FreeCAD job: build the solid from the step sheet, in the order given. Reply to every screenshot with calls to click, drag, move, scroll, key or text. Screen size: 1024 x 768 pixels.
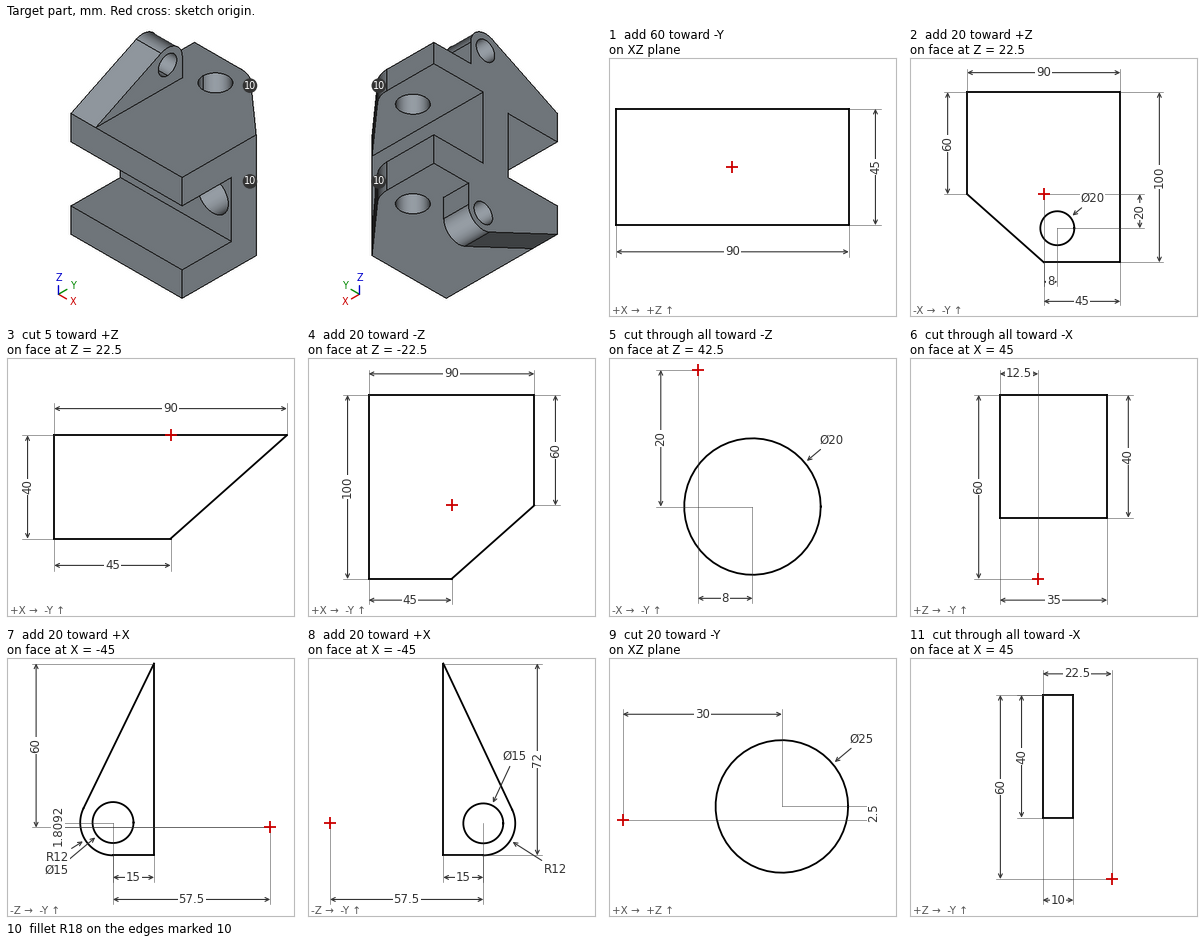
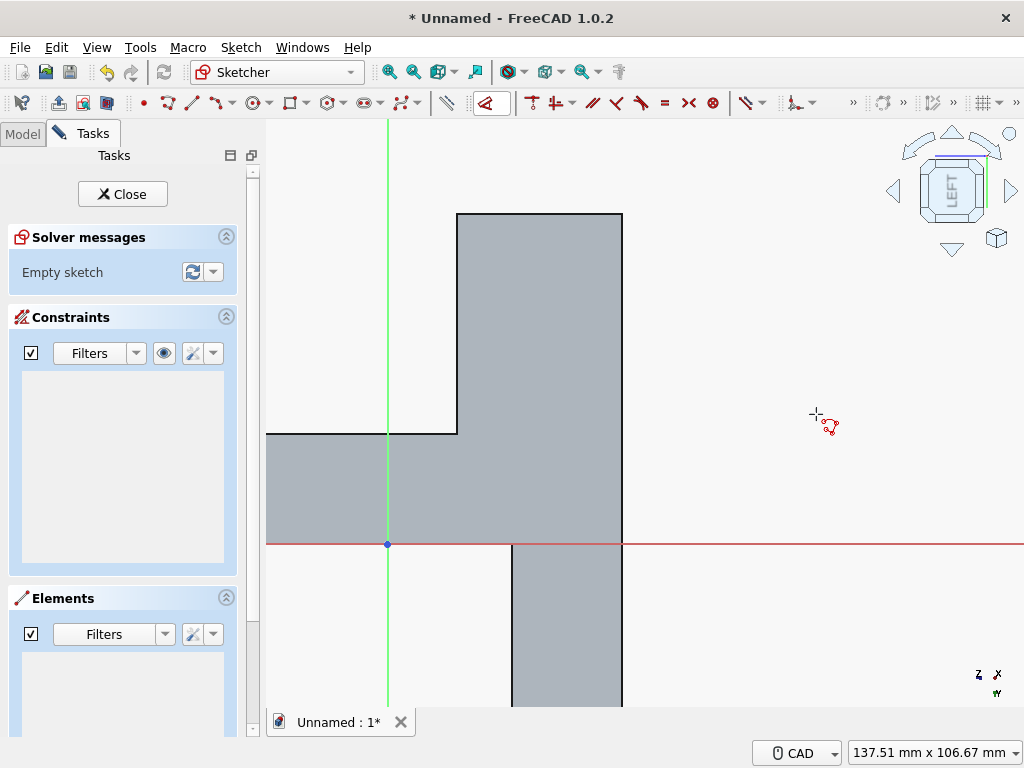
click(765, 516)
click(622, 214)
click(622, 611)
click(705, 611)
right_click(705, 611)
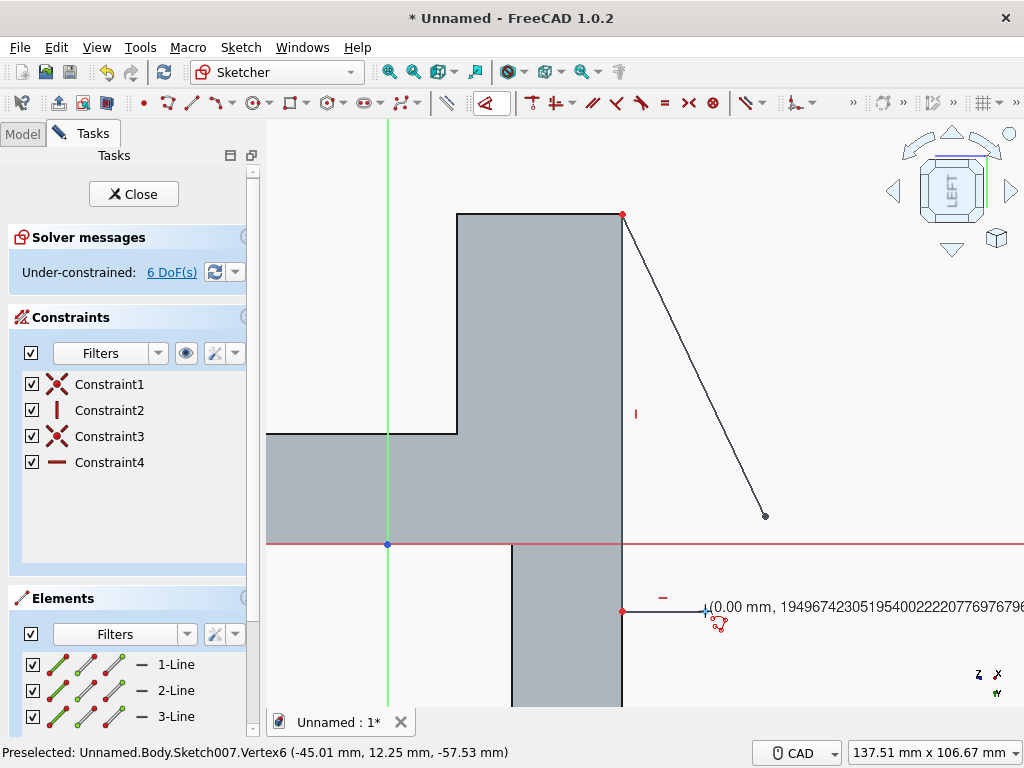
key(g)
key(3)
key(a)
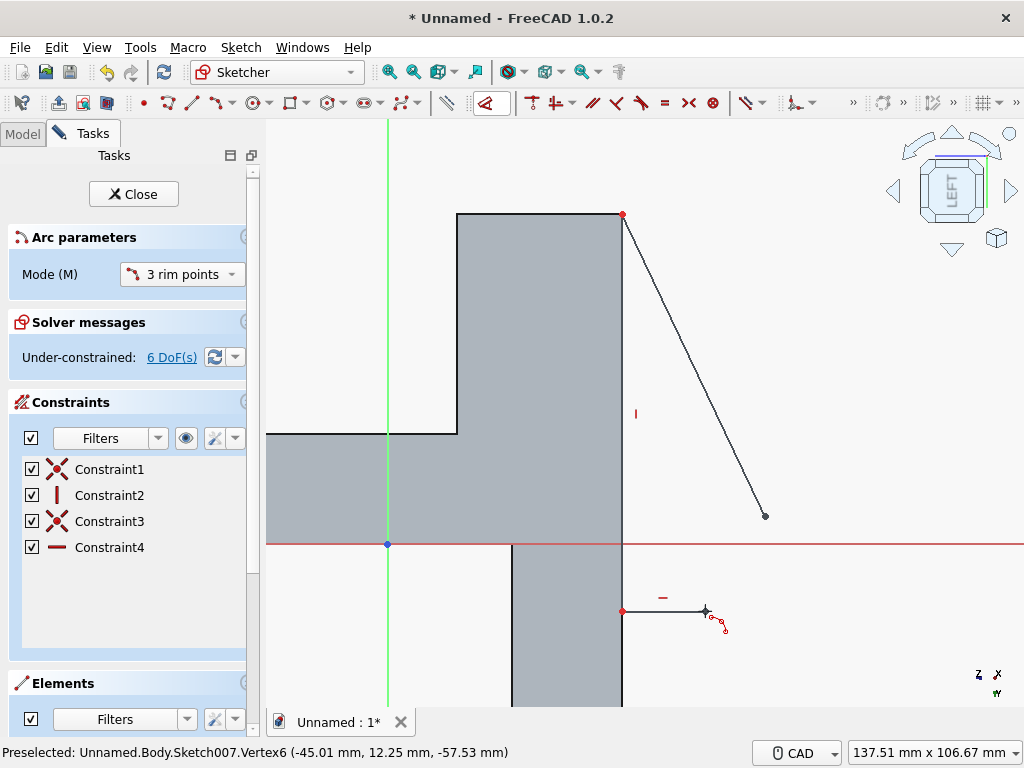
click(705, 612)
click(765, 517)
click(761, 580)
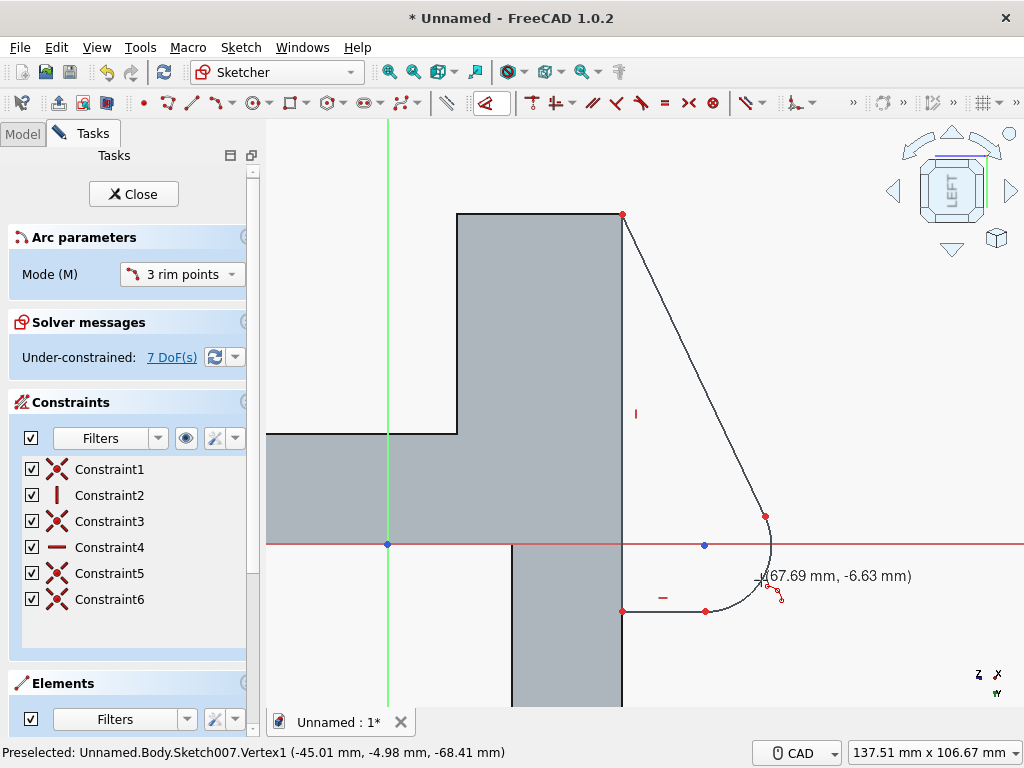
click(254, 104)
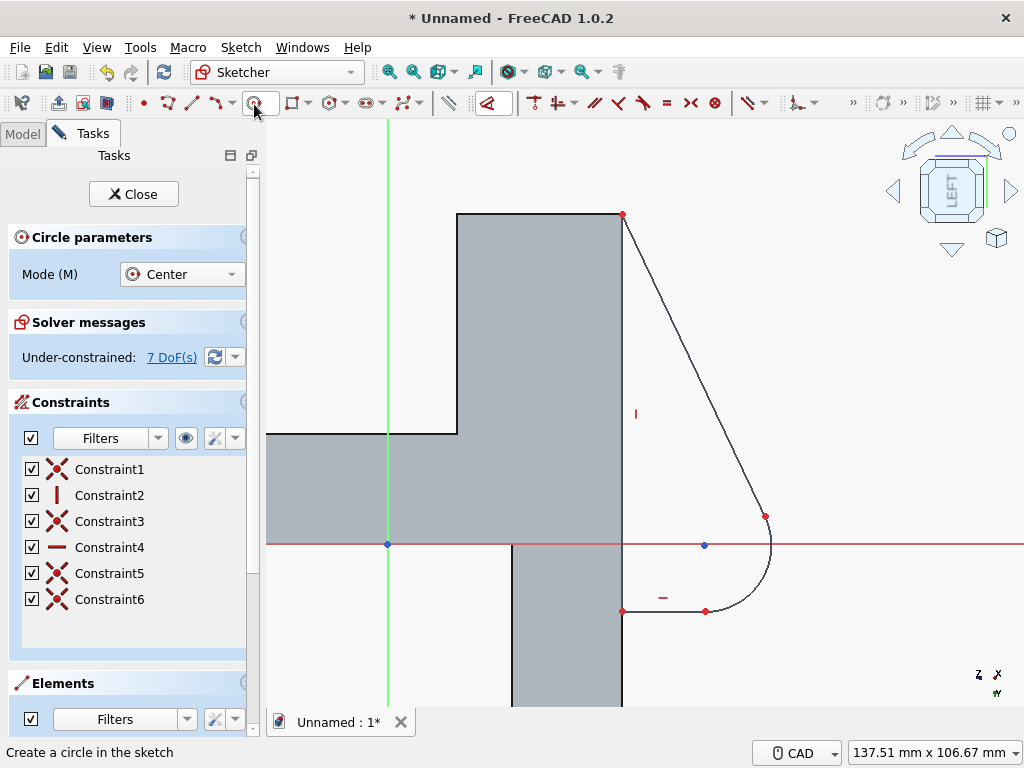
click(705, 544)
move(734, 515)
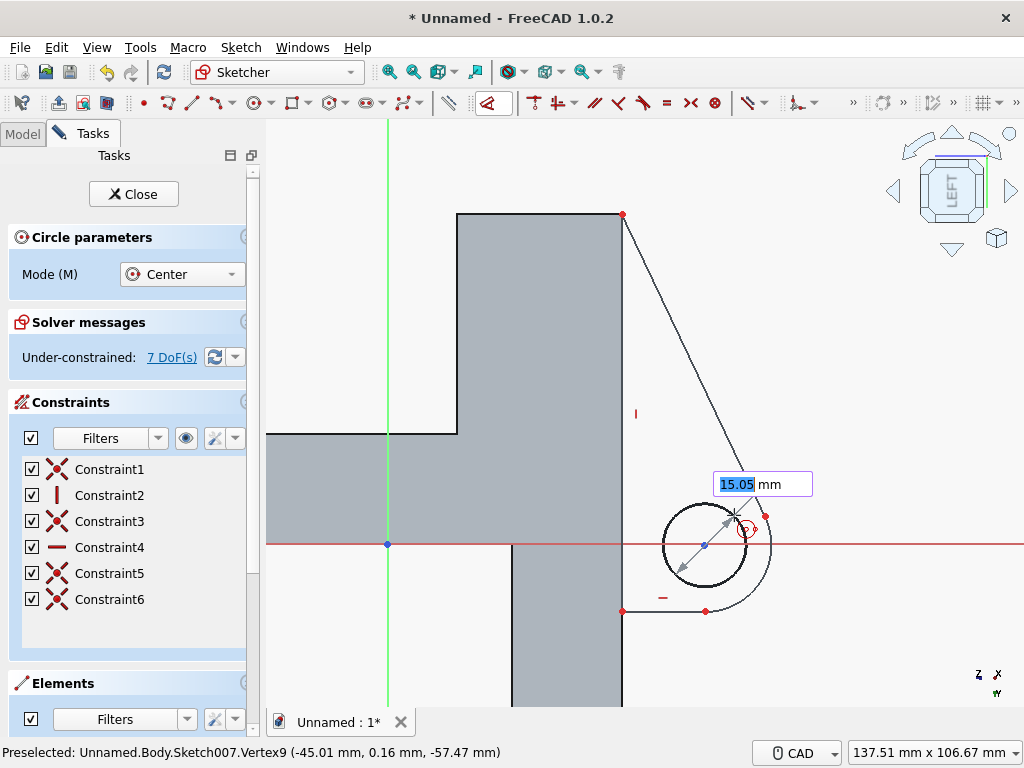
text(15)
key(Return)
key(Escape)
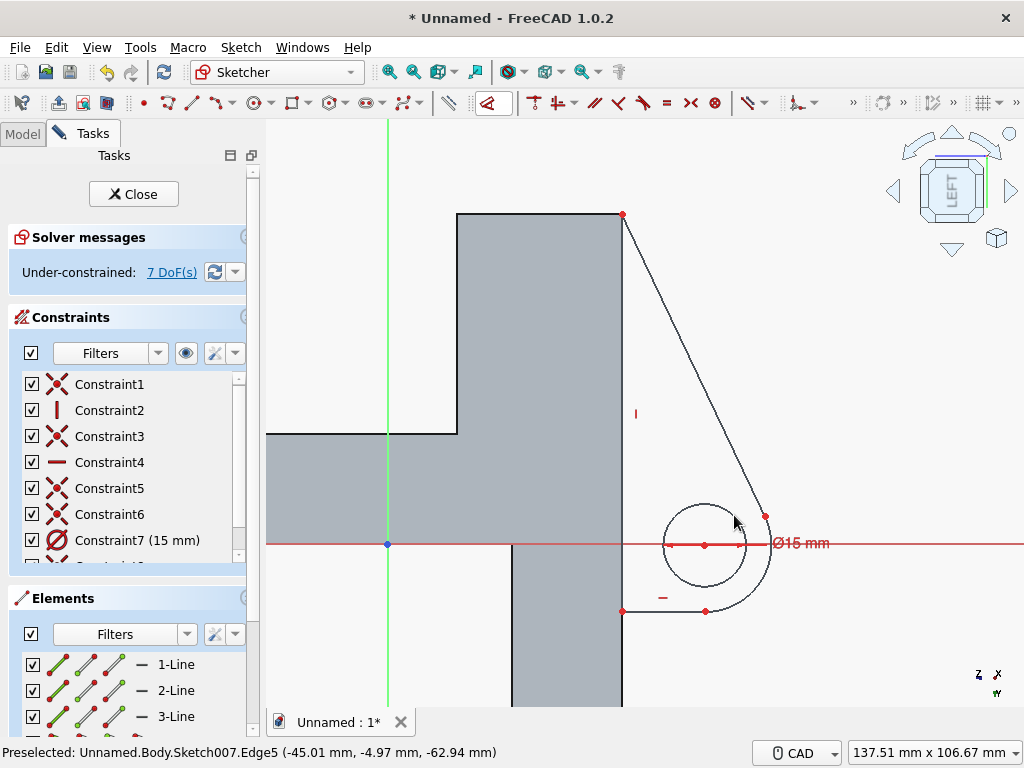
click(722, 426)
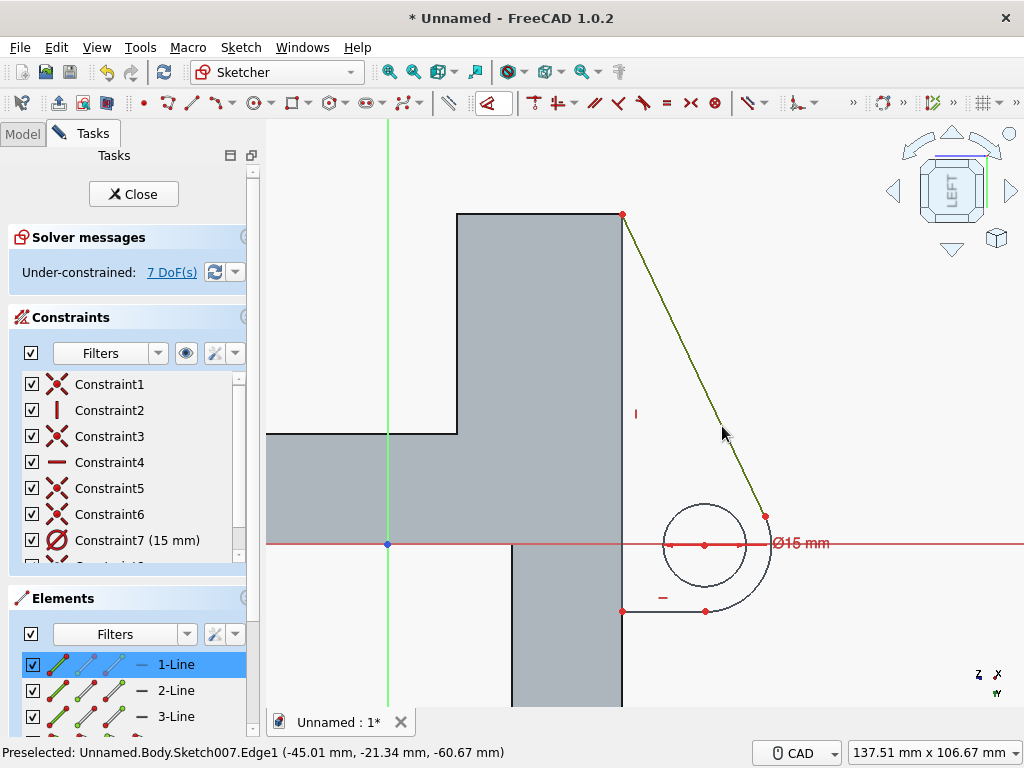
click(743, 600)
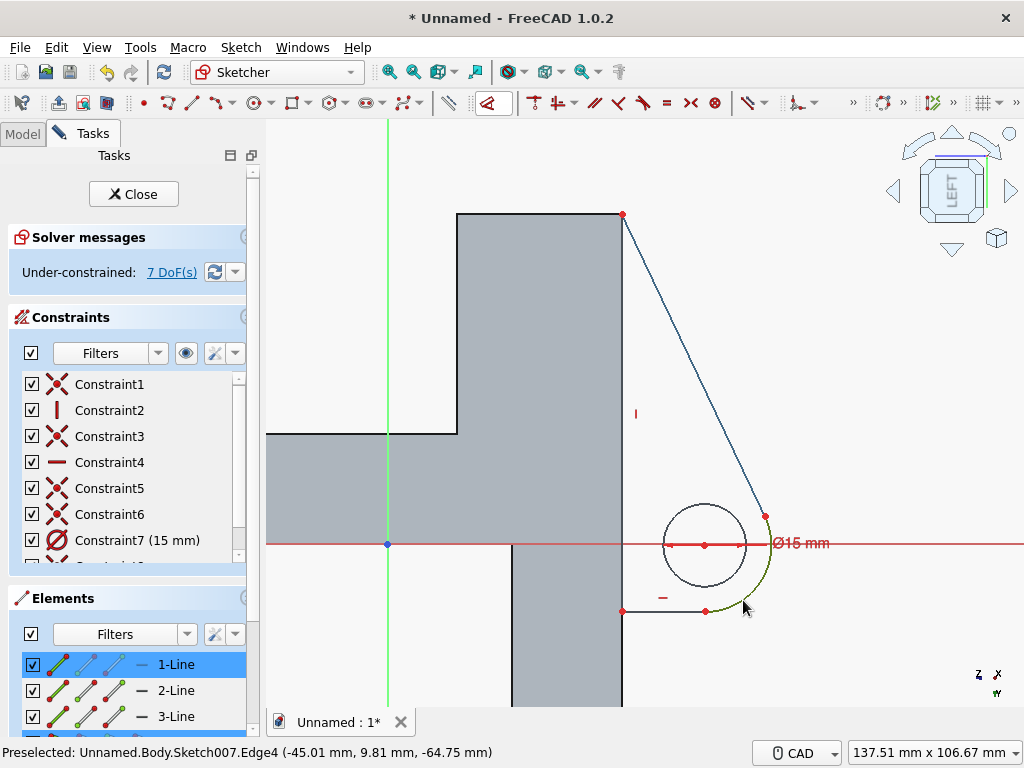
click(644, 104)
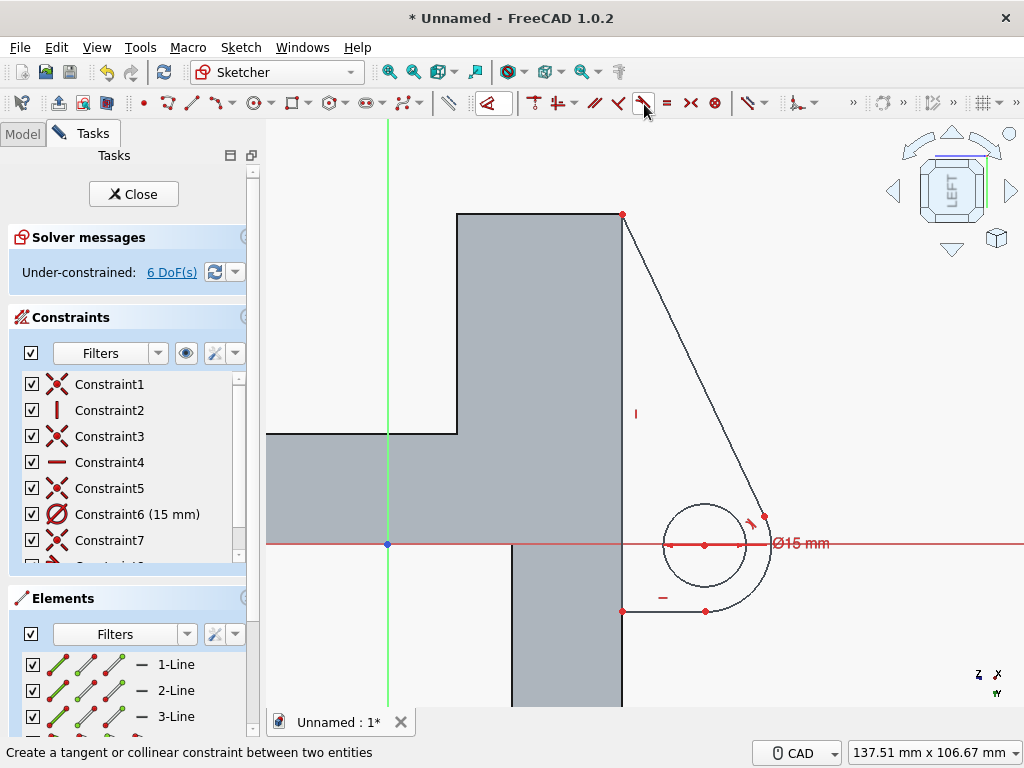
click(647, 612)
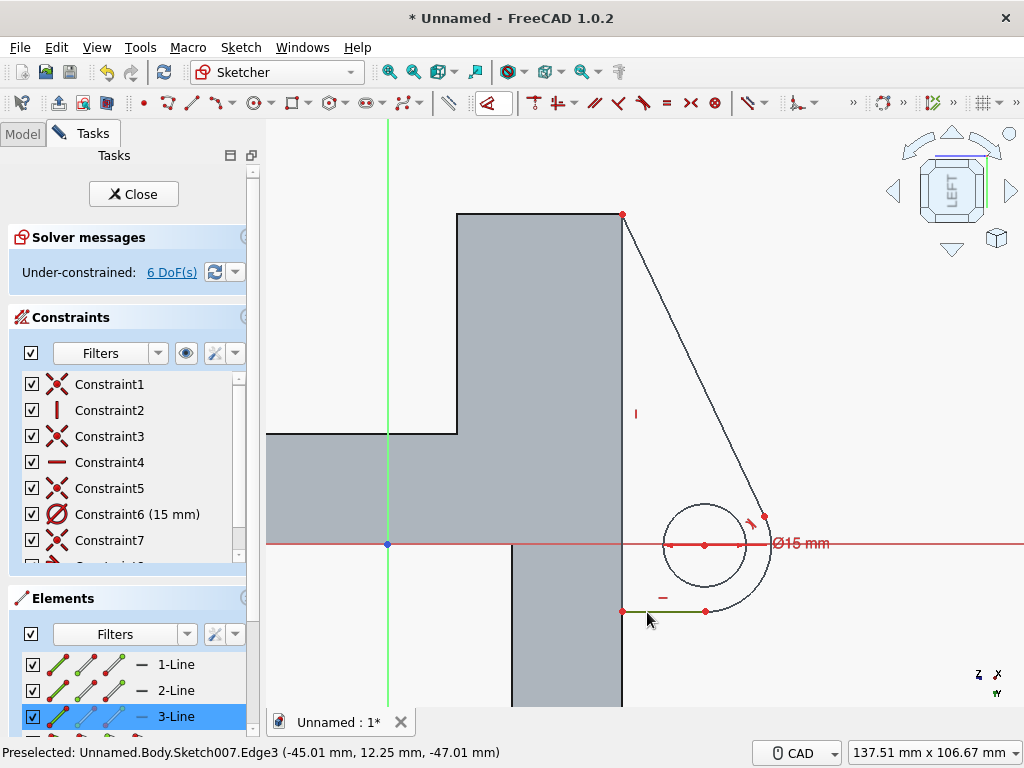
click(743, 600)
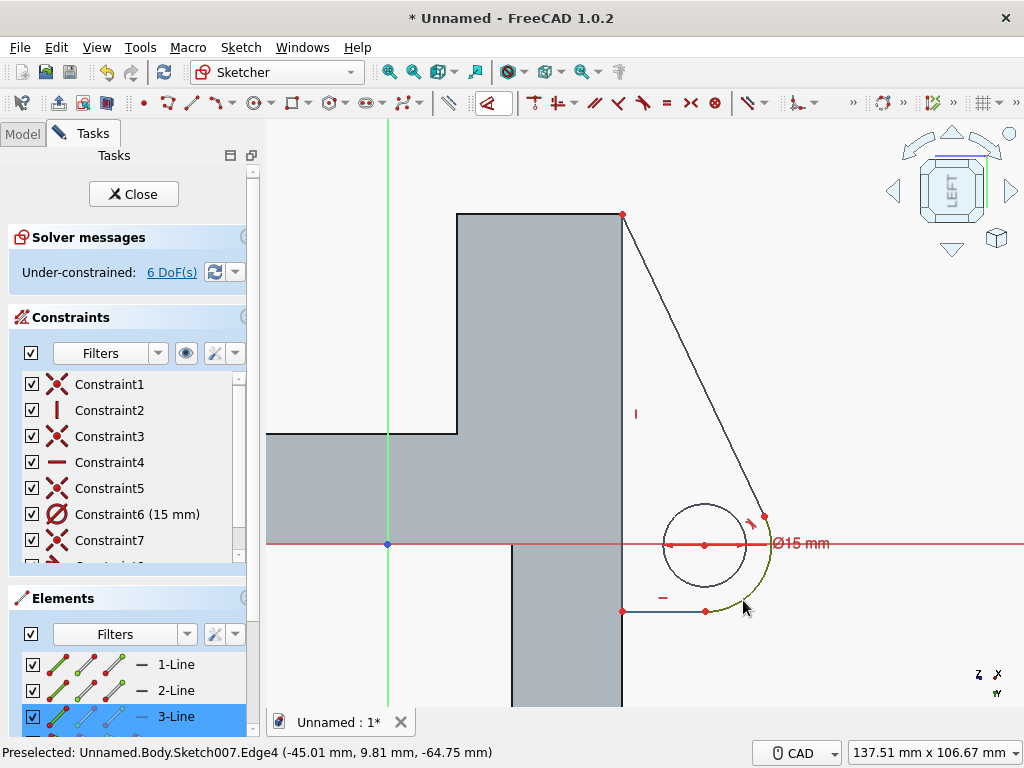
key(t)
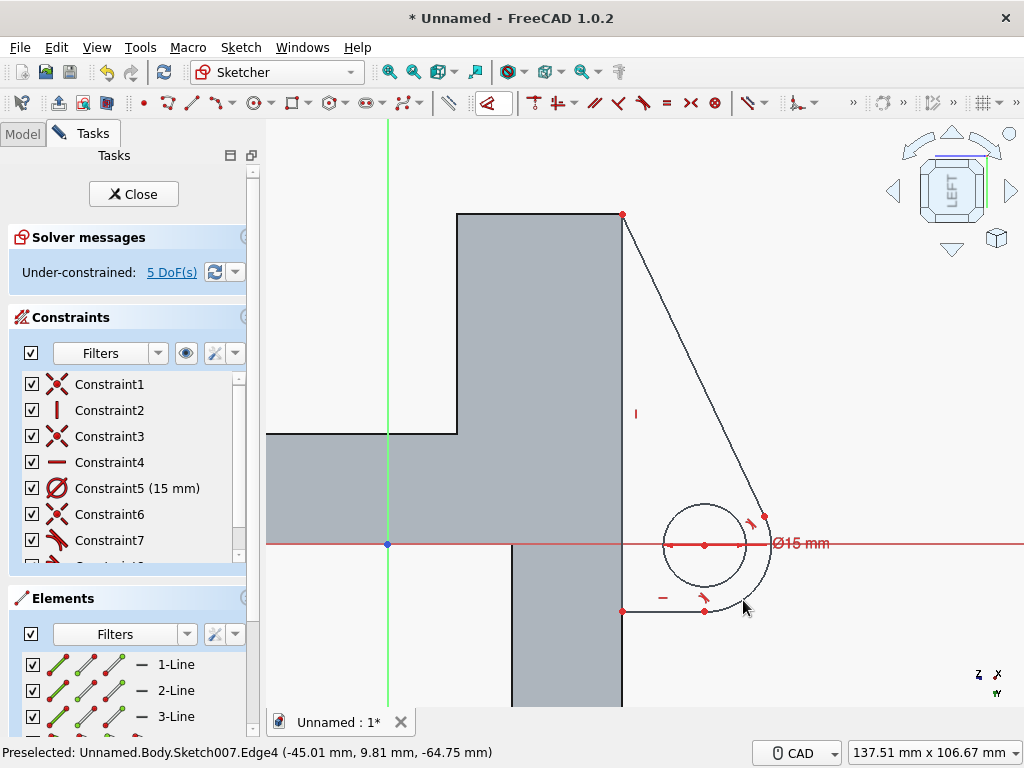
click(705, 545)